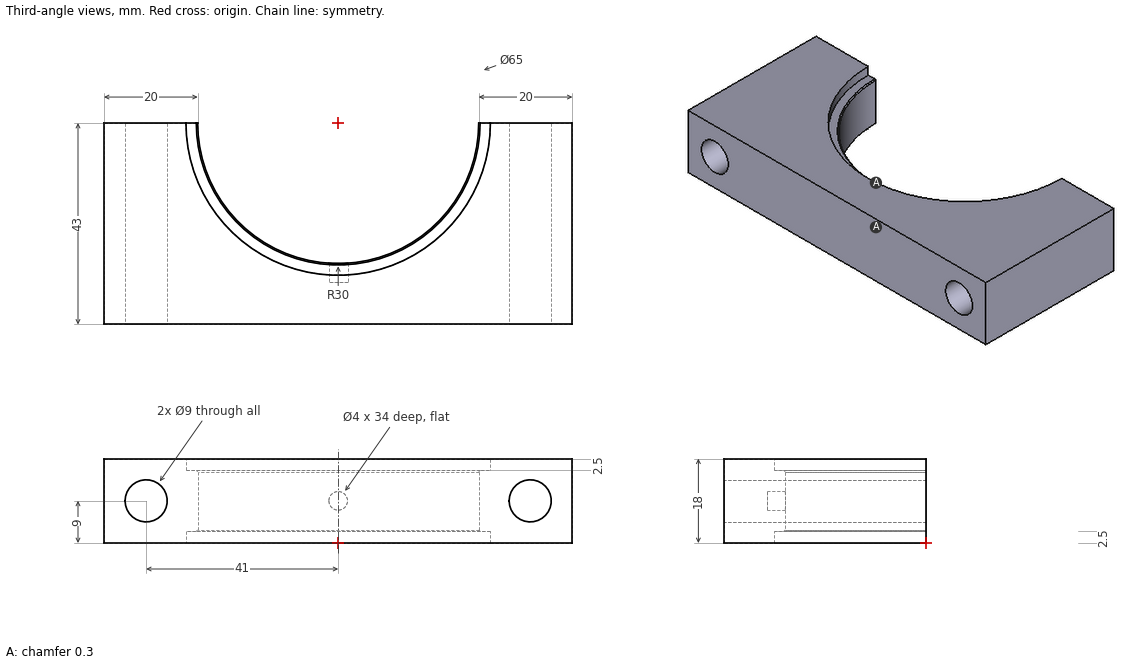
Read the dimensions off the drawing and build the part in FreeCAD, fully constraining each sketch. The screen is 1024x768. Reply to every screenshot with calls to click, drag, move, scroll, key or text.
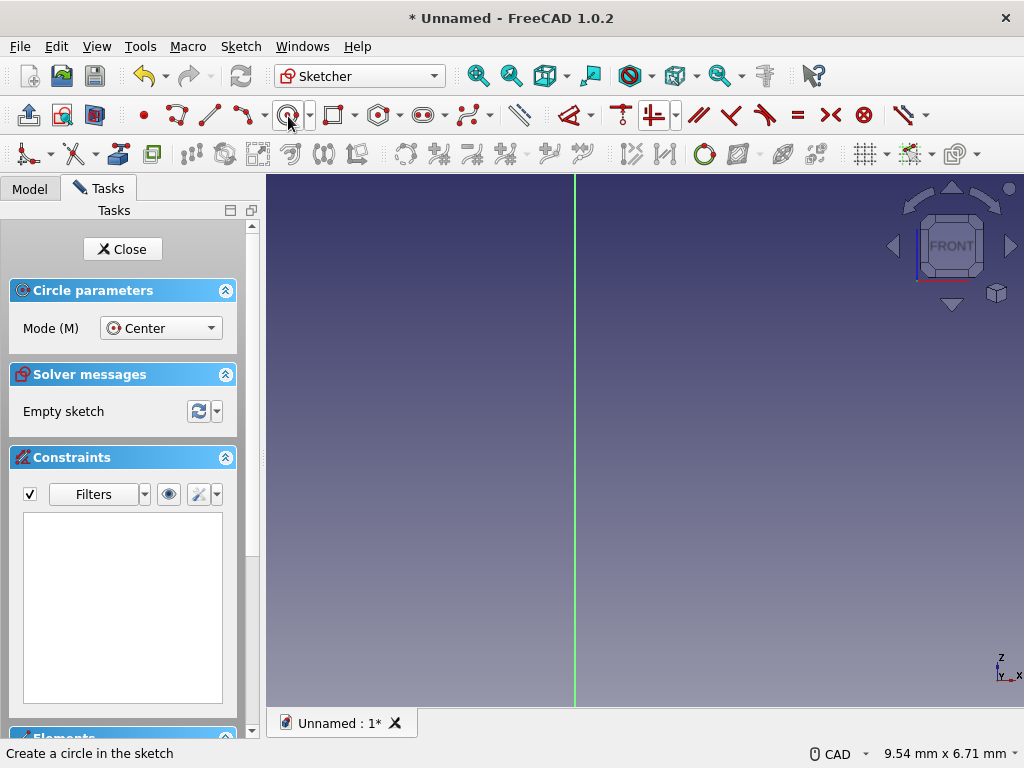
click(575, 440)
move(688, 328)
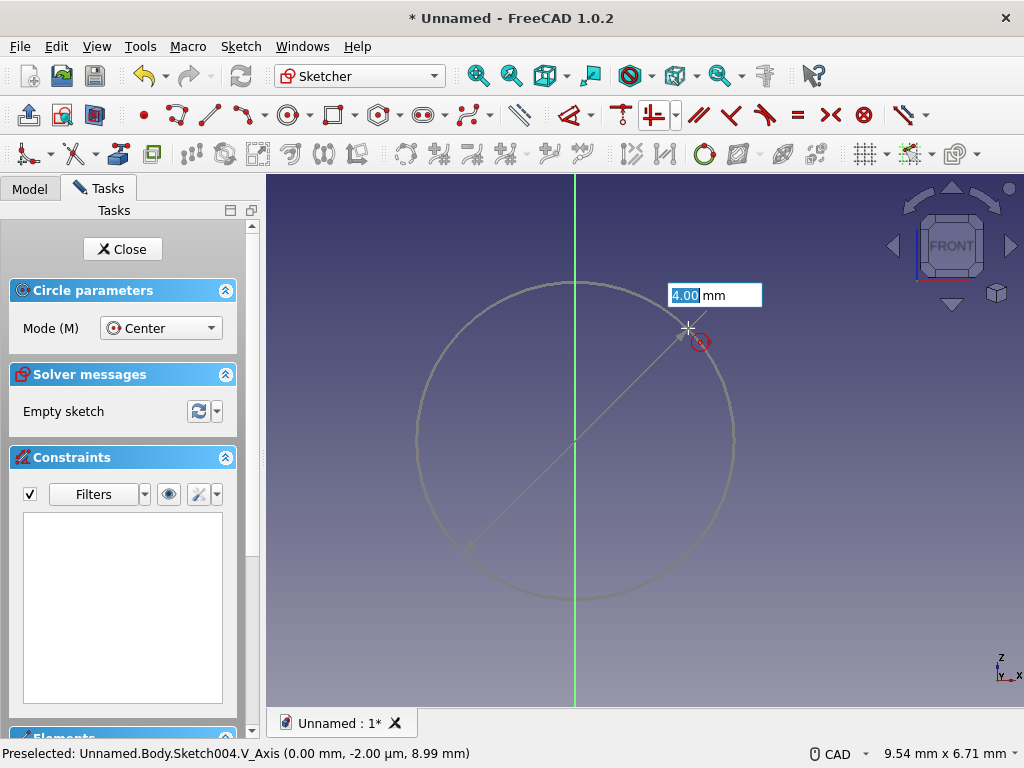
text(4)
key(Return)
key(Escape)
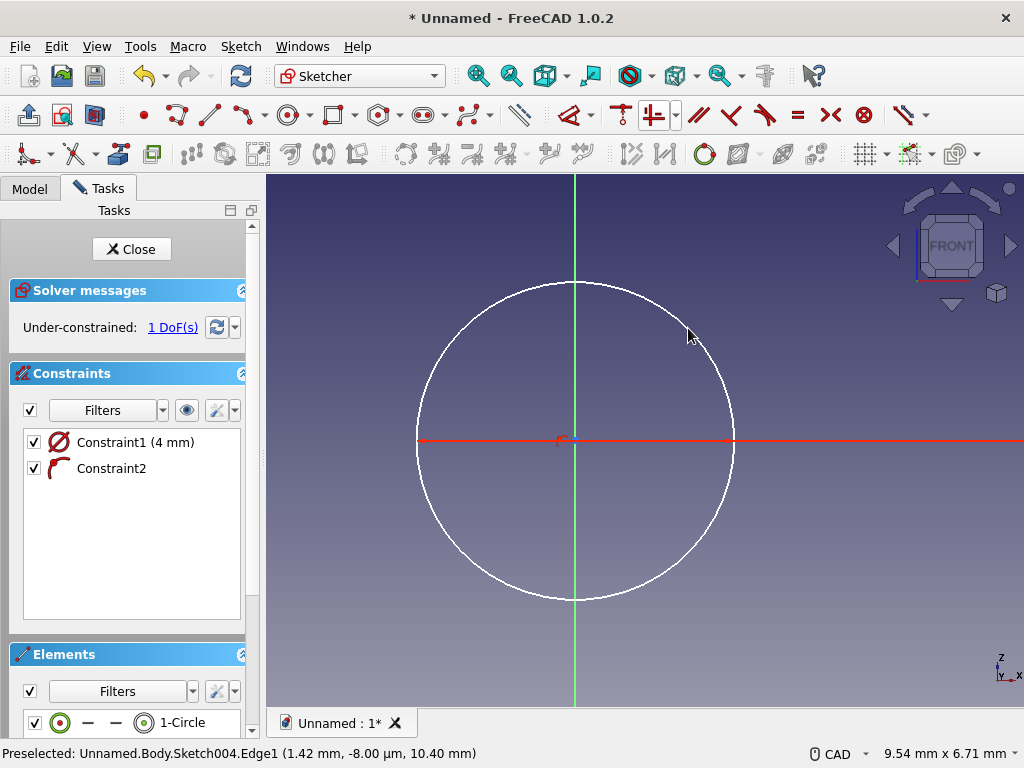
click(568, 116)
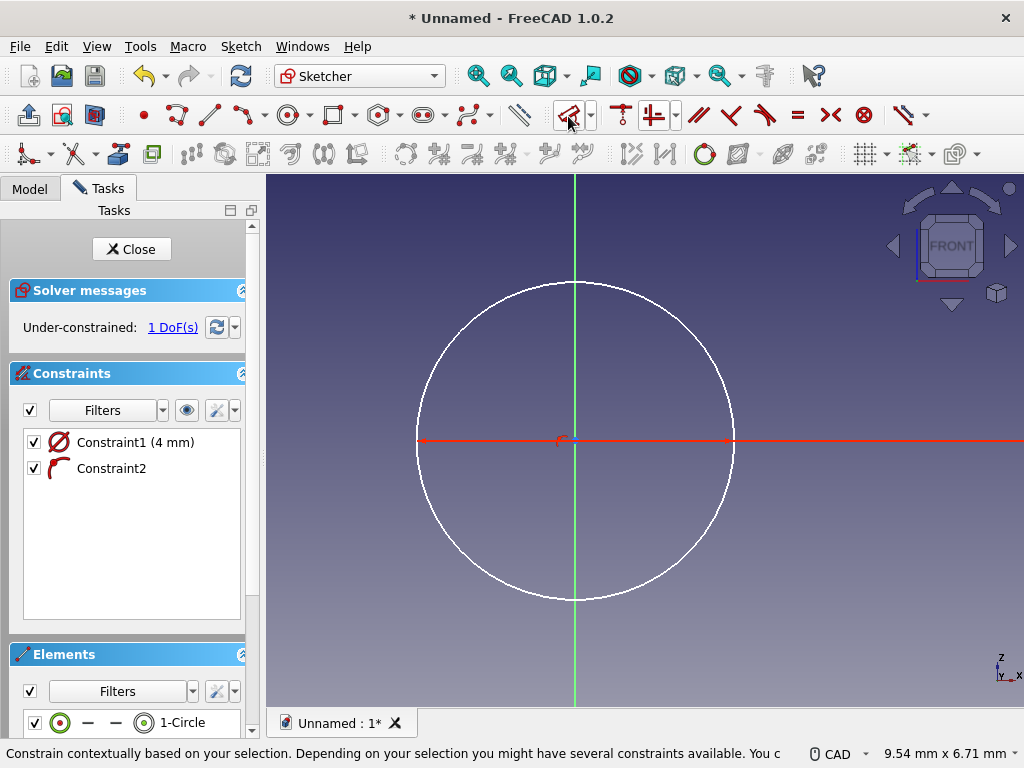
click(575, 441)
click(609, 560)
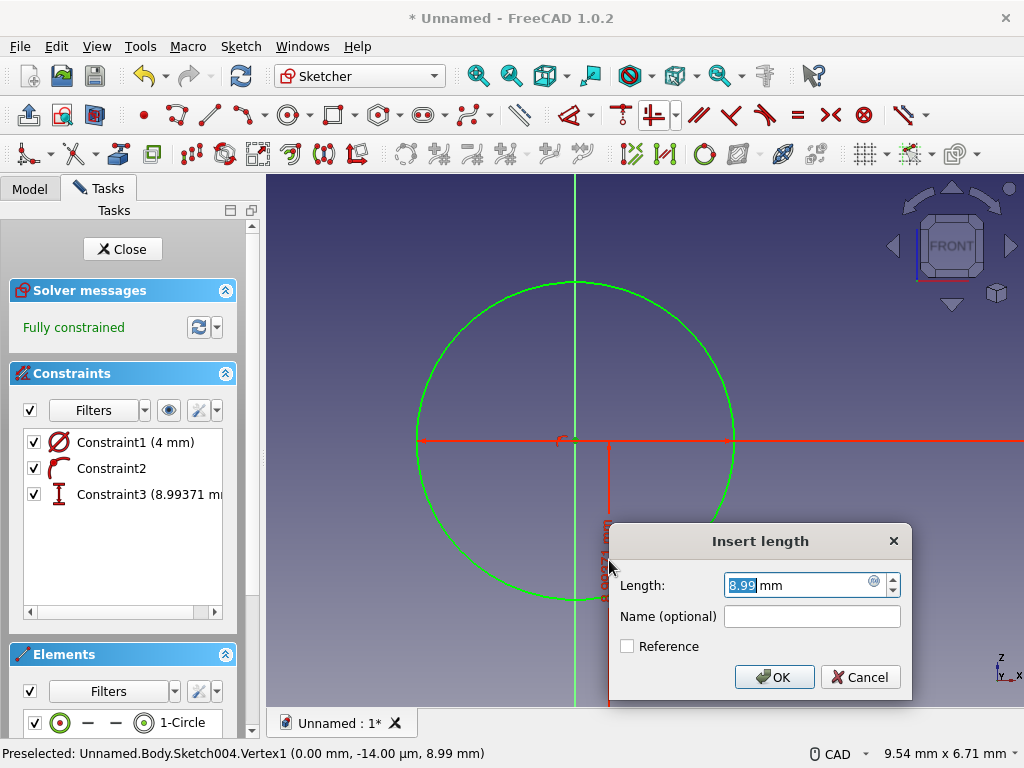
text(9)
key(Return)
key(Escape)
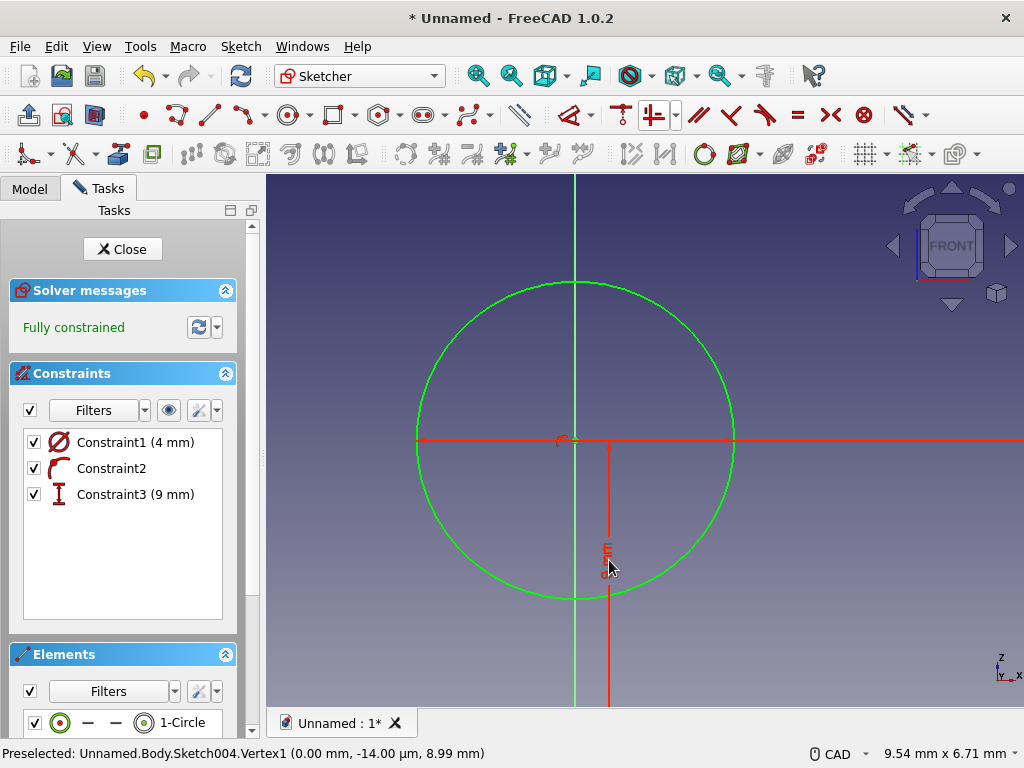
click(123, 249)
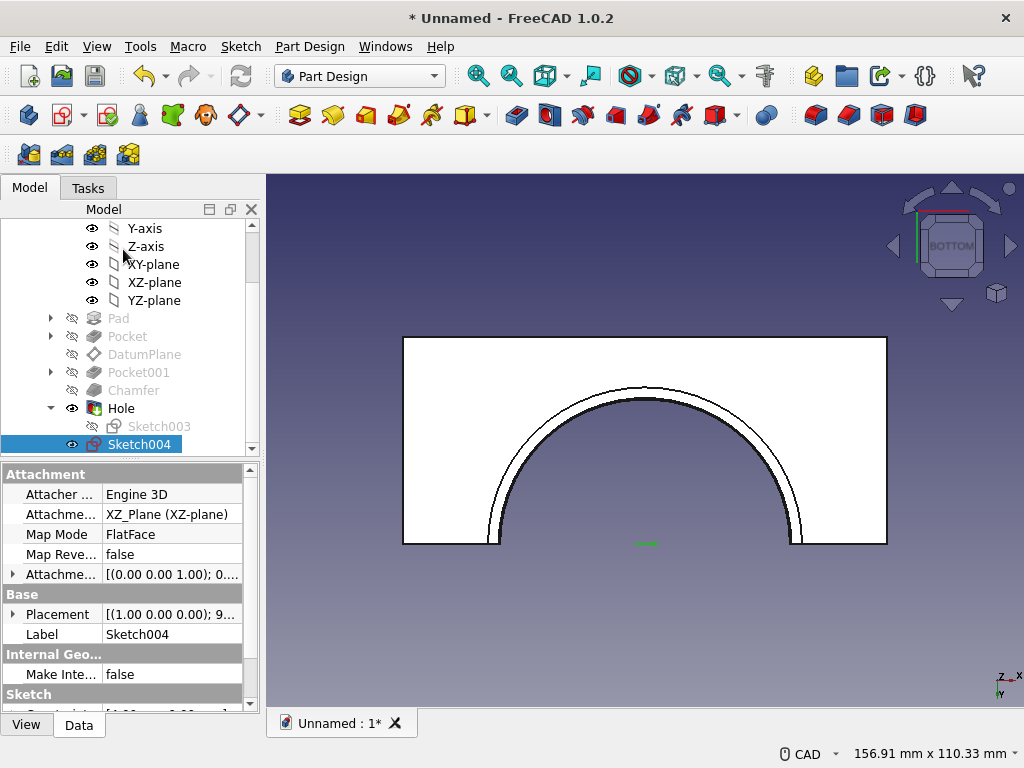
click(550, 116)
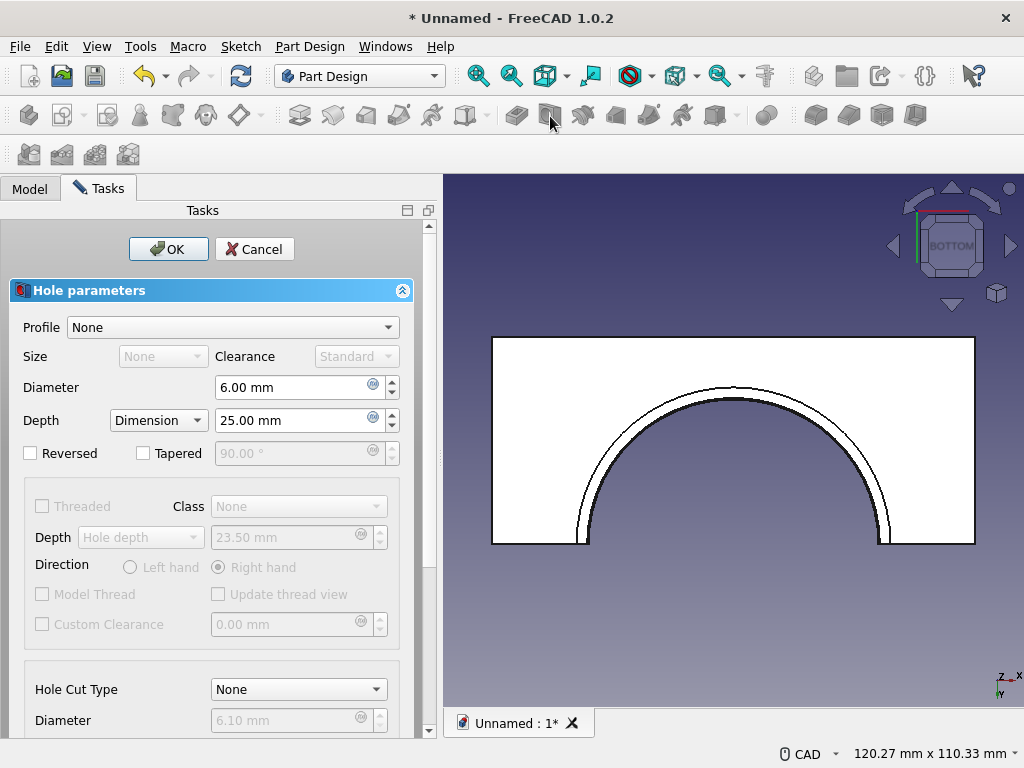
triple_click(300, 388)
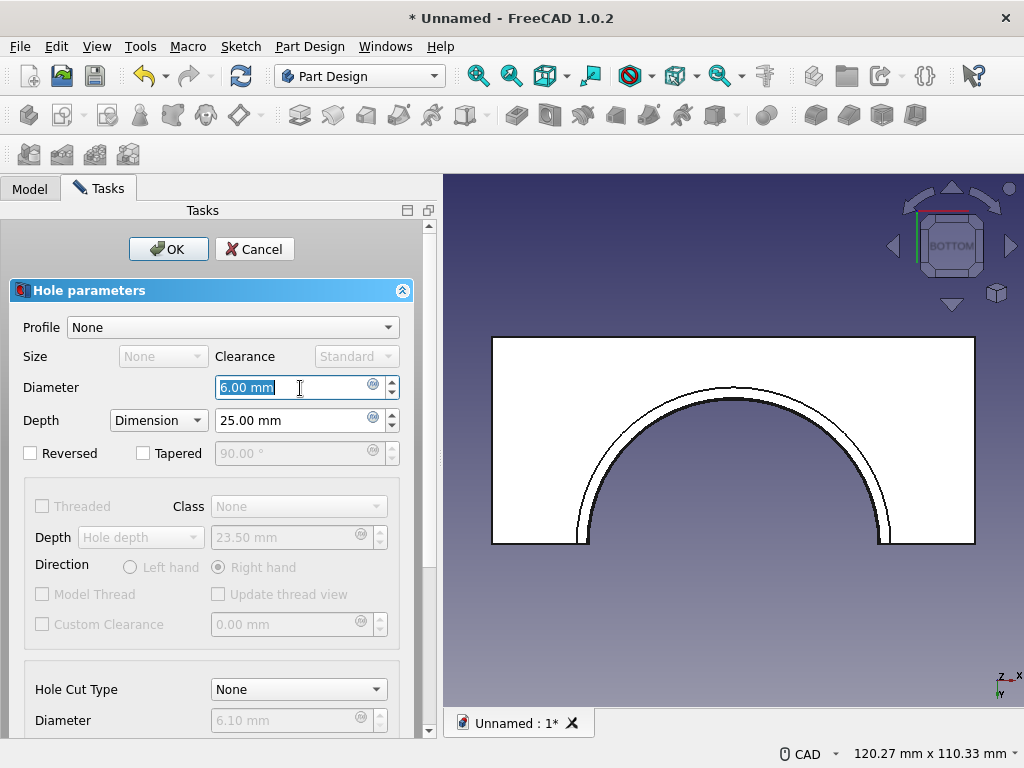
text(4)
key(Tab)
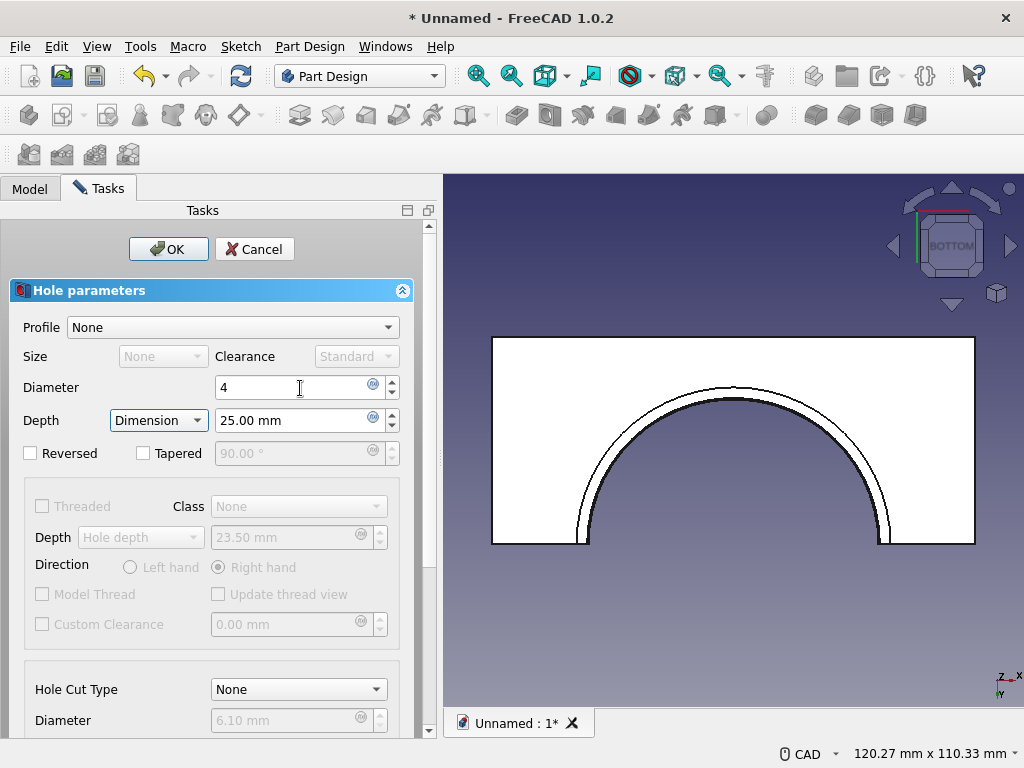
triple_click(300, 420)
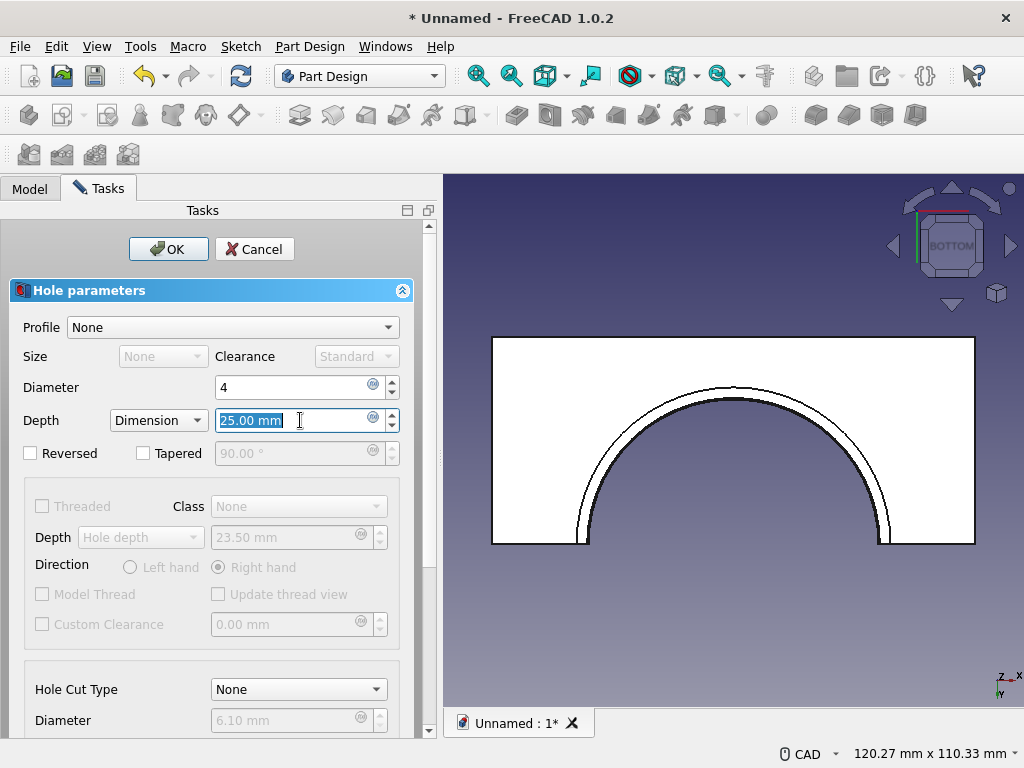
text(34)
key(Tab)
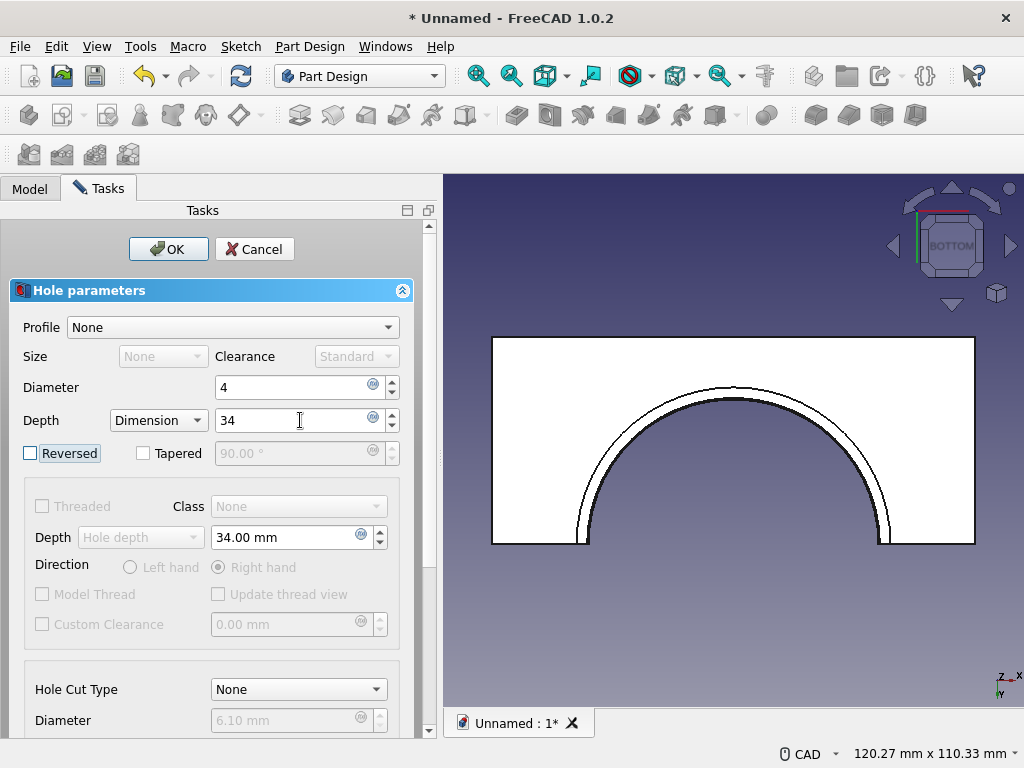
click(31, 453)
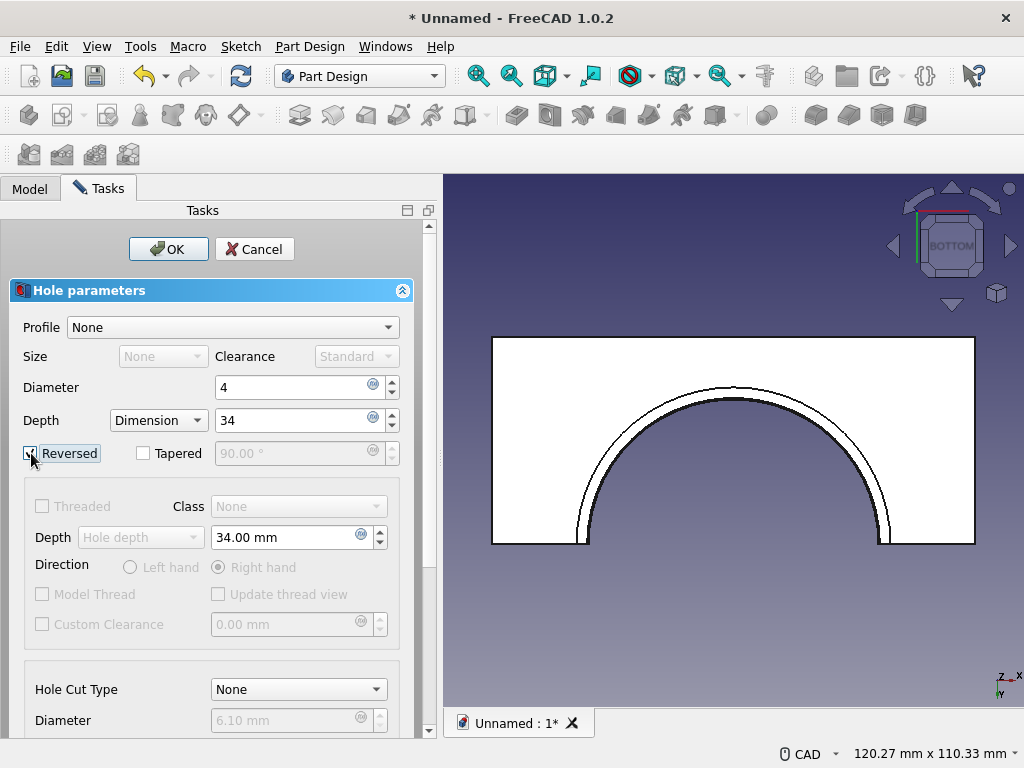
scroll(429, 479, down, 4)